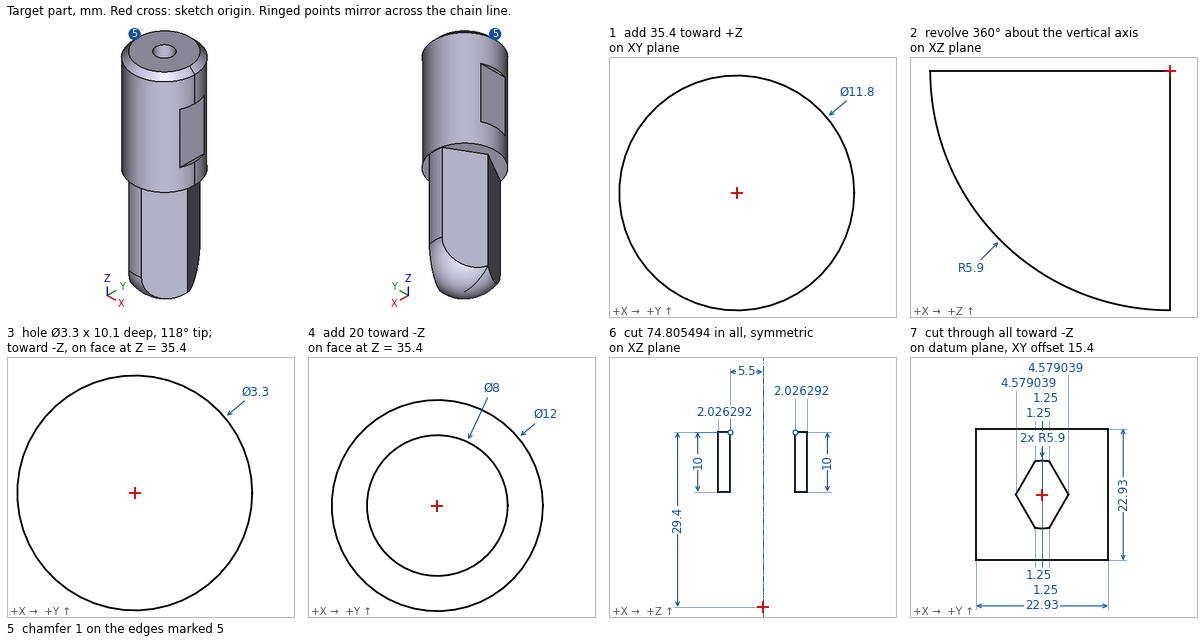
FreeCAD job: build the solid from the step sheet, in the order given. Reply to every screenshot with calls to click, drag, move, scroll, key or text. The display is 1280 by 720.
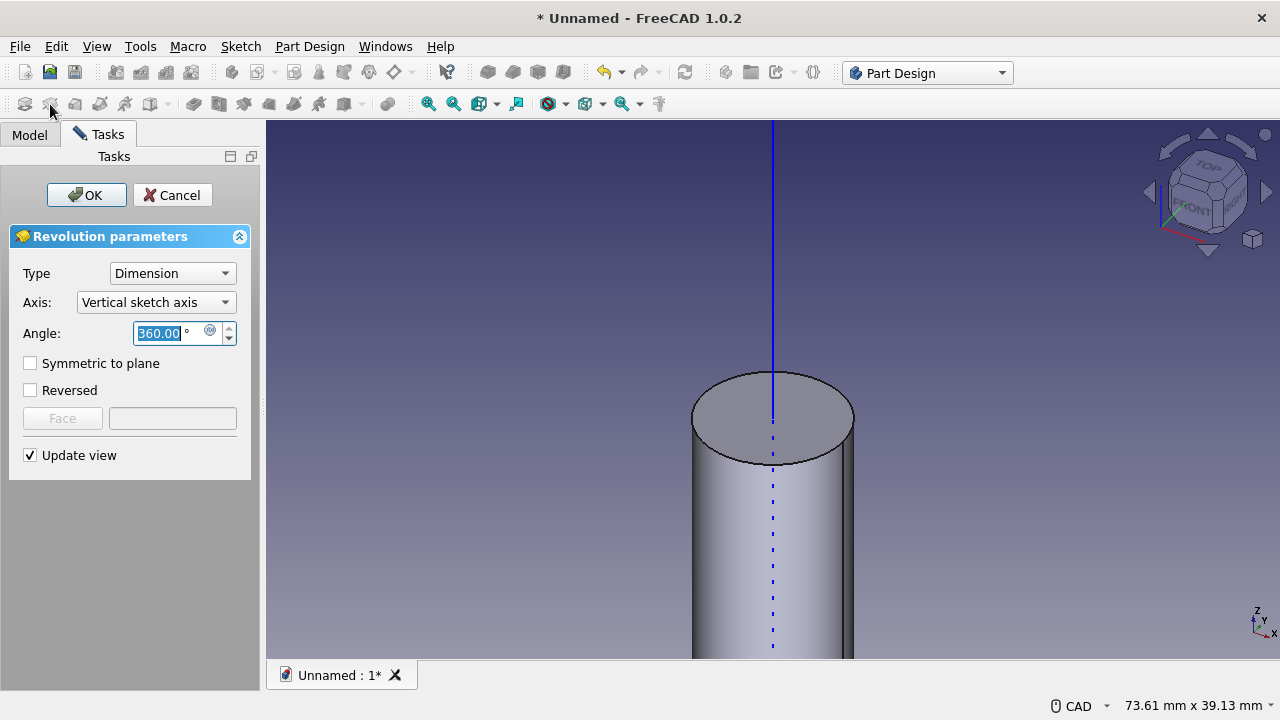
click(87, 195)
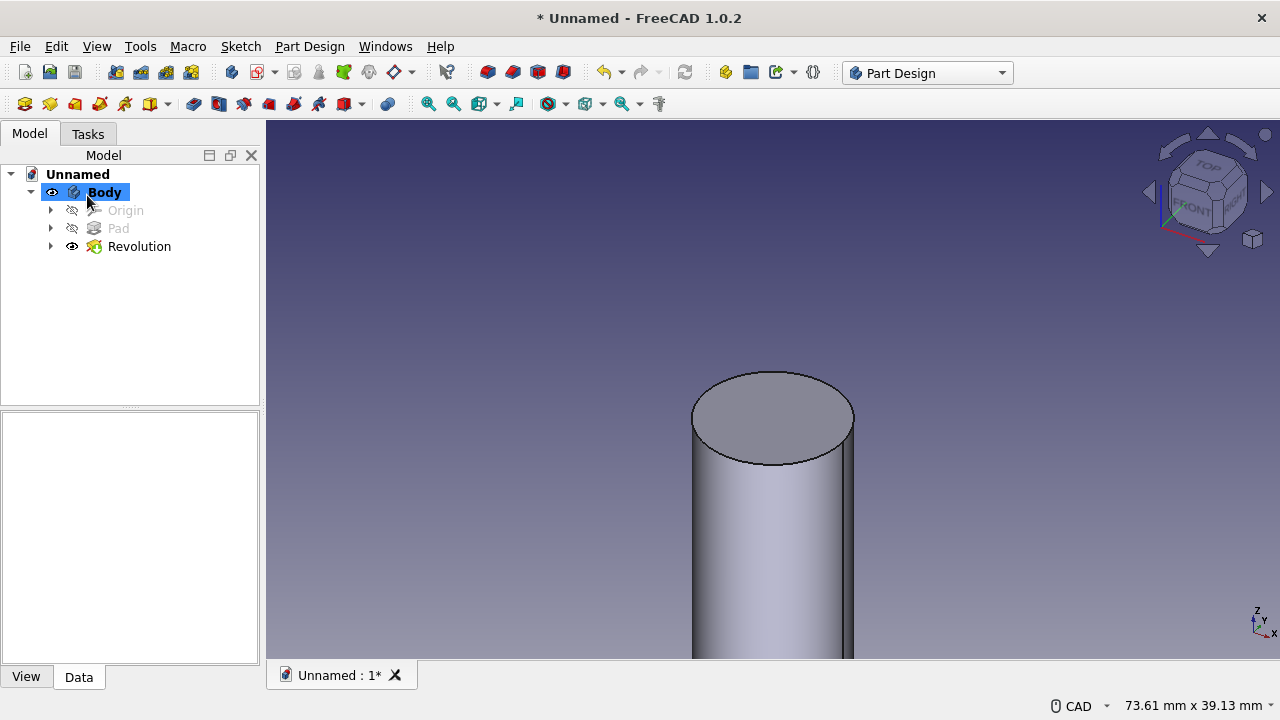
key(v)
key(f)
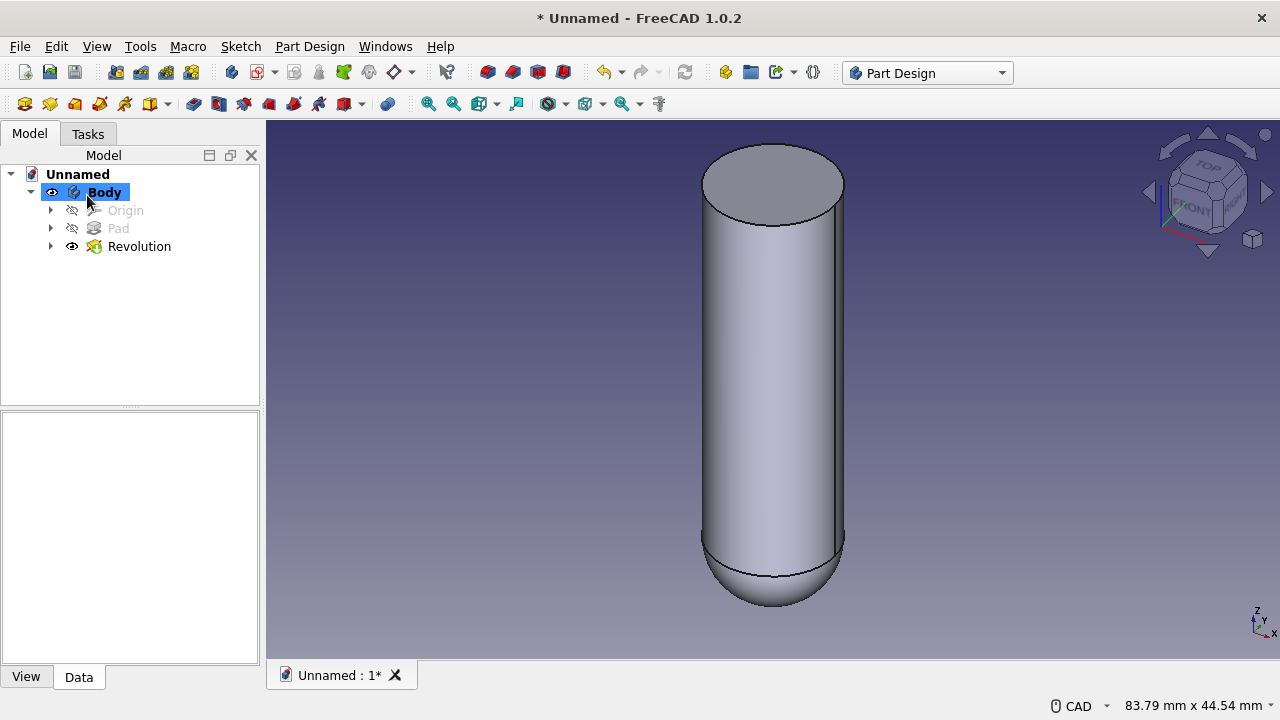
click(773, 184)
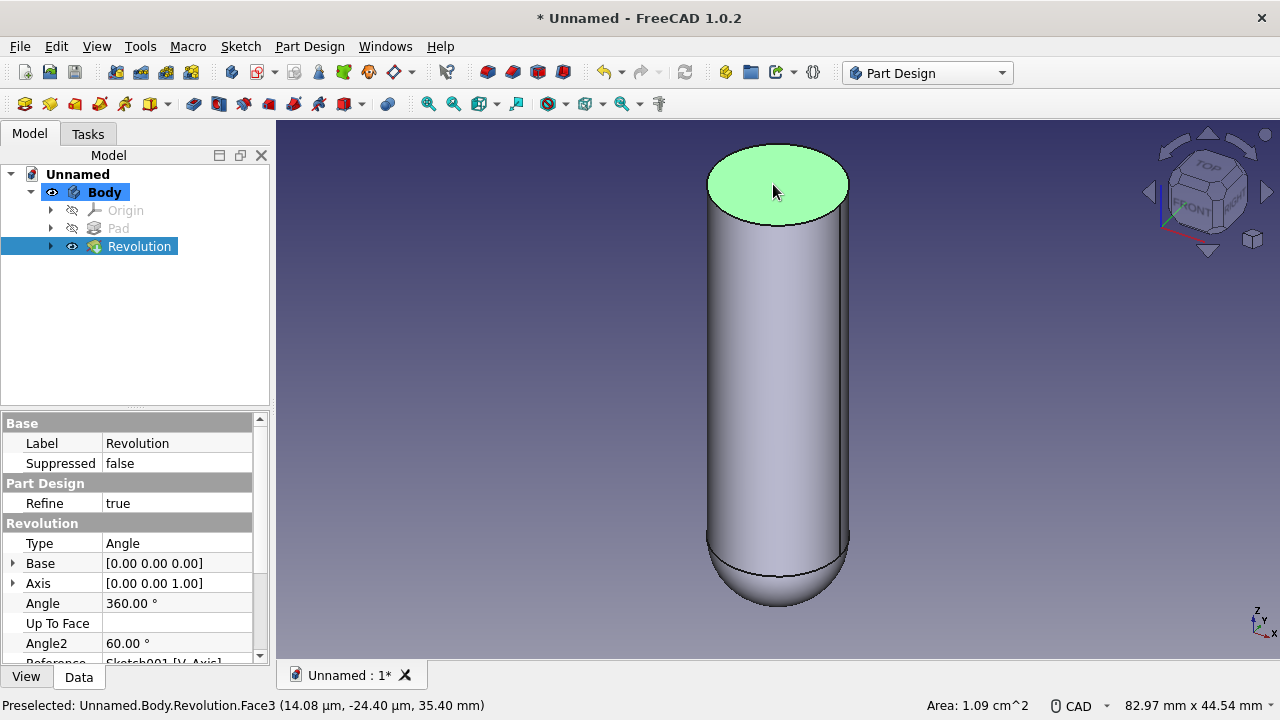
click(256, 72)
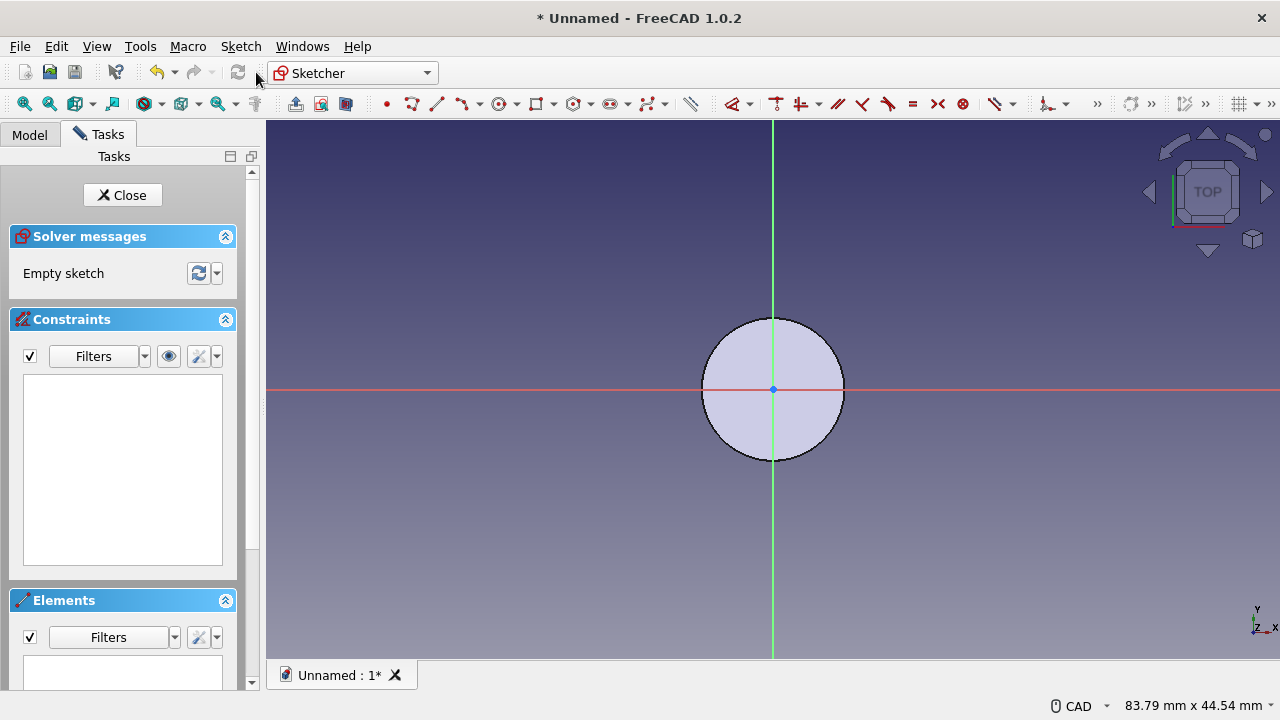
scroll(782, 390, up, 11)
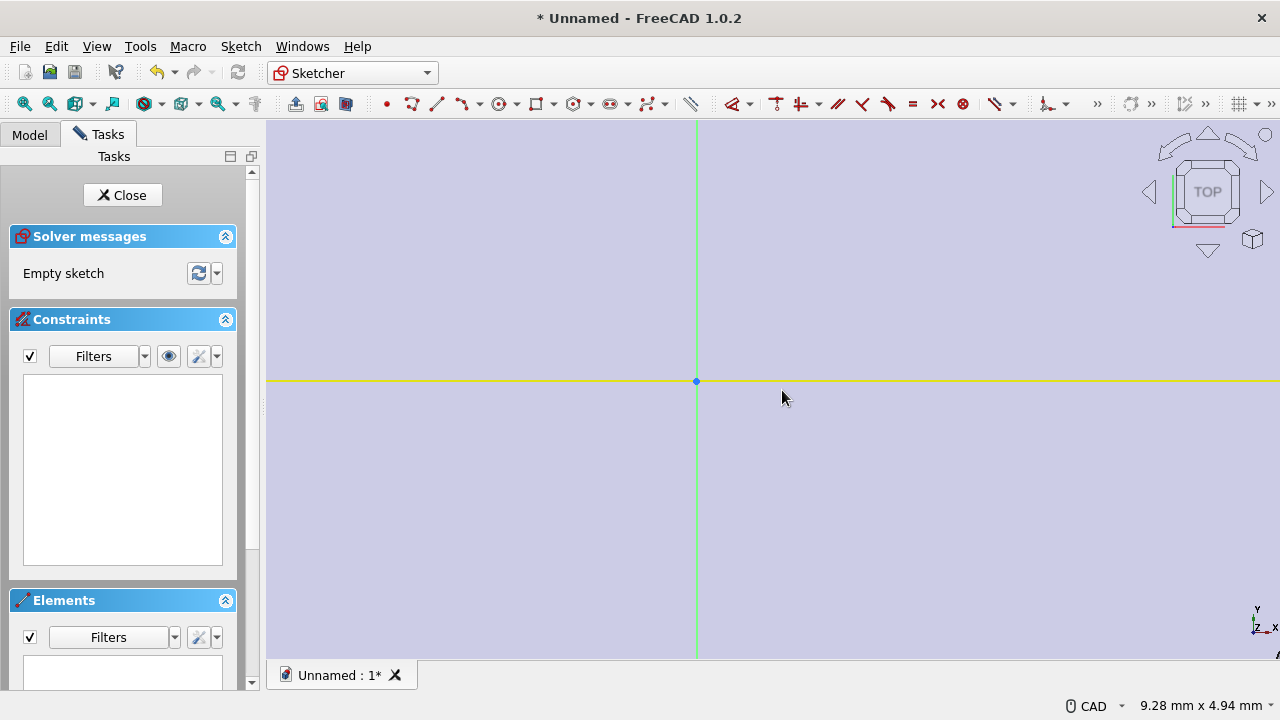
key(g)
key(c)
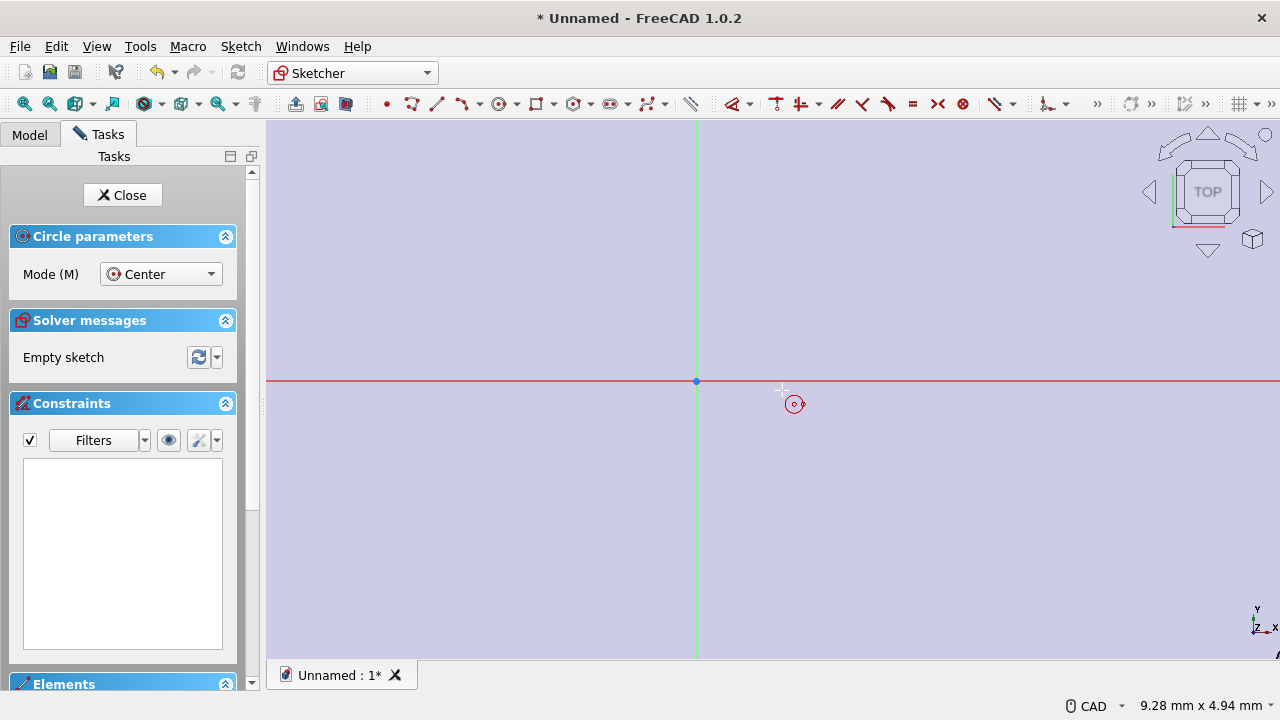
click(697, 381)
move(824, 254)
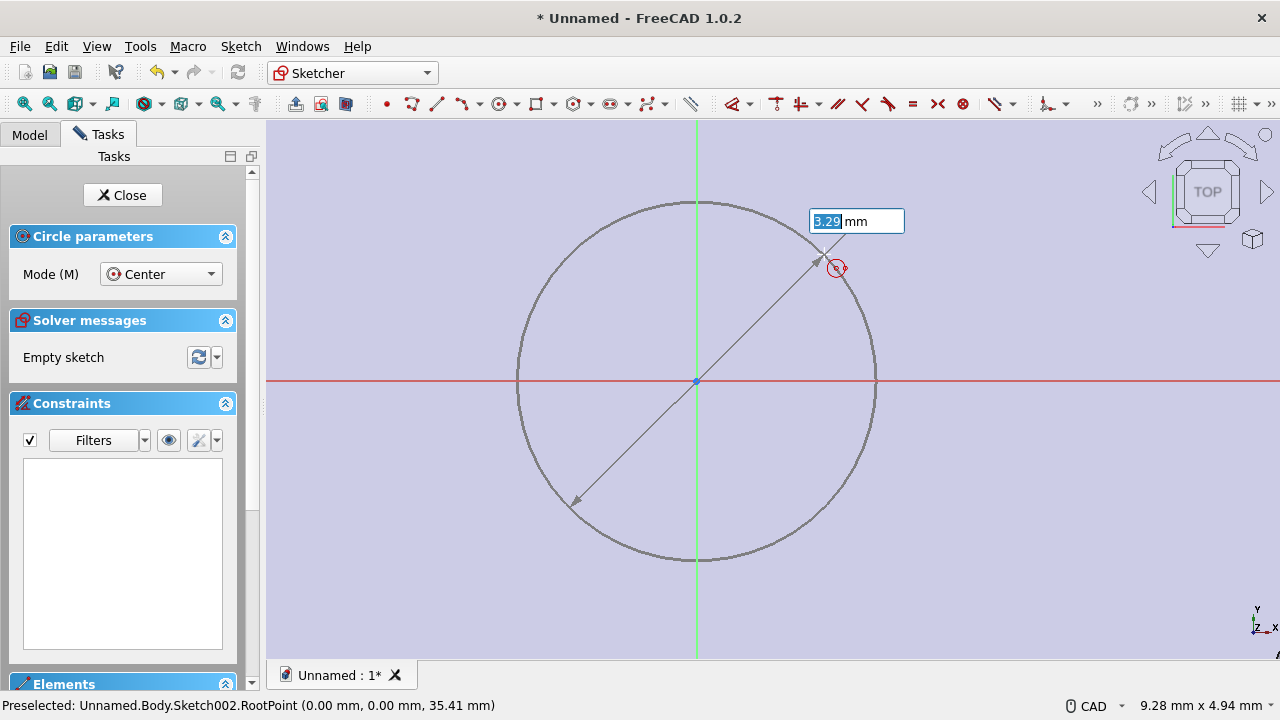
text(3.3)
key(Return)
key(Escape)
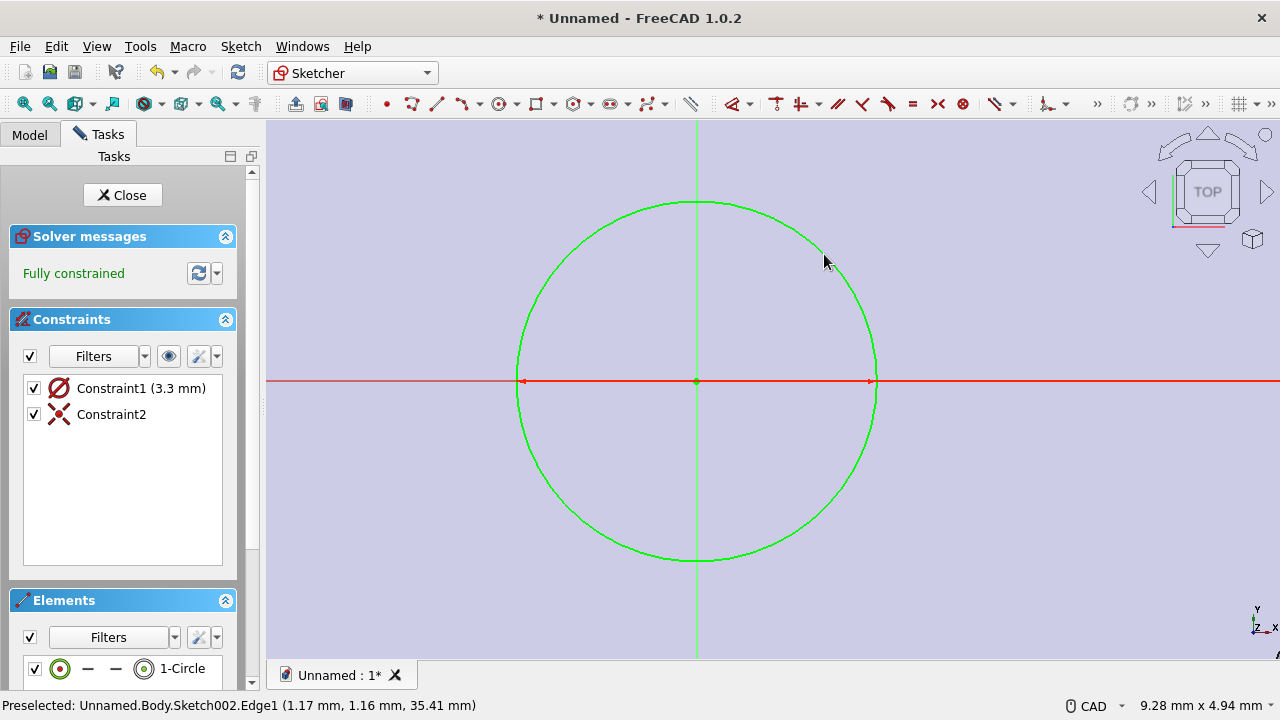
click(123, 195)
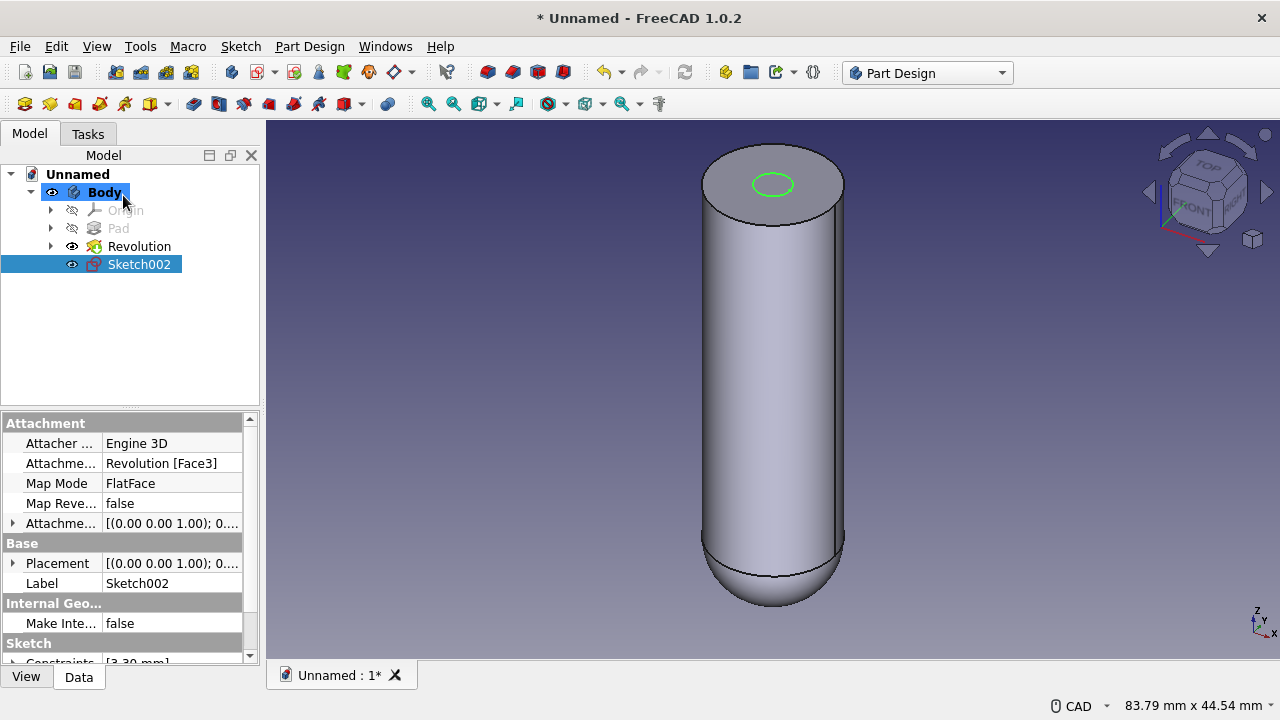
click(219, 104)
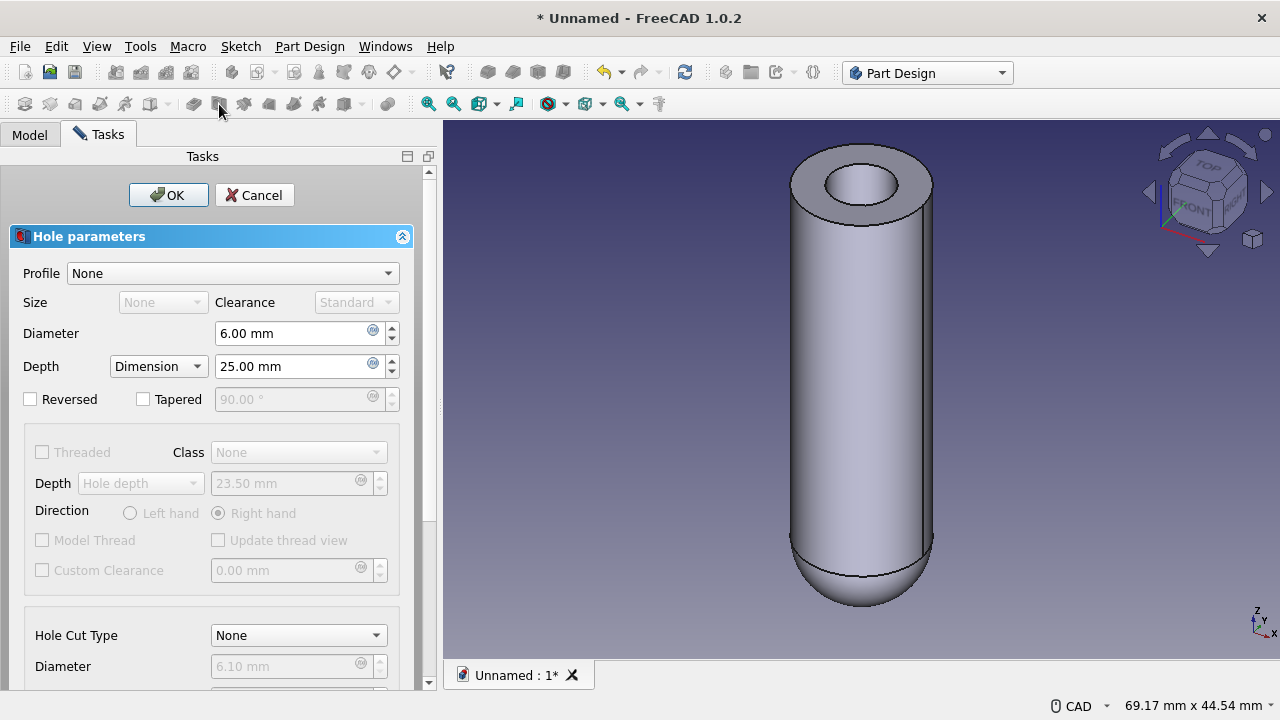
triple_click(300, 334)